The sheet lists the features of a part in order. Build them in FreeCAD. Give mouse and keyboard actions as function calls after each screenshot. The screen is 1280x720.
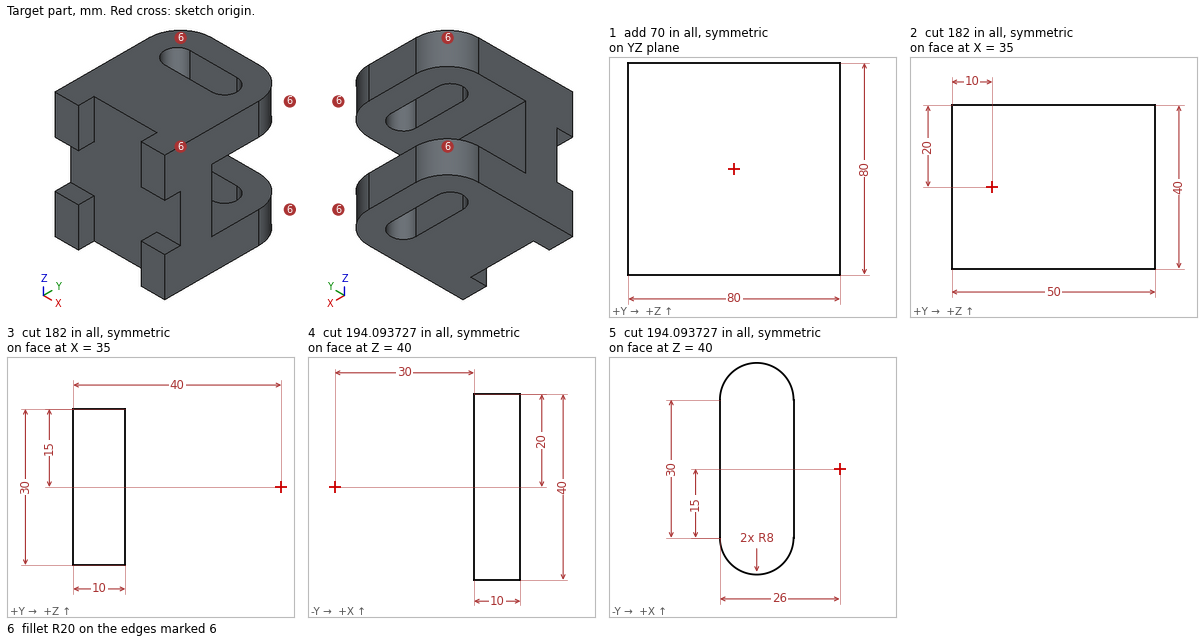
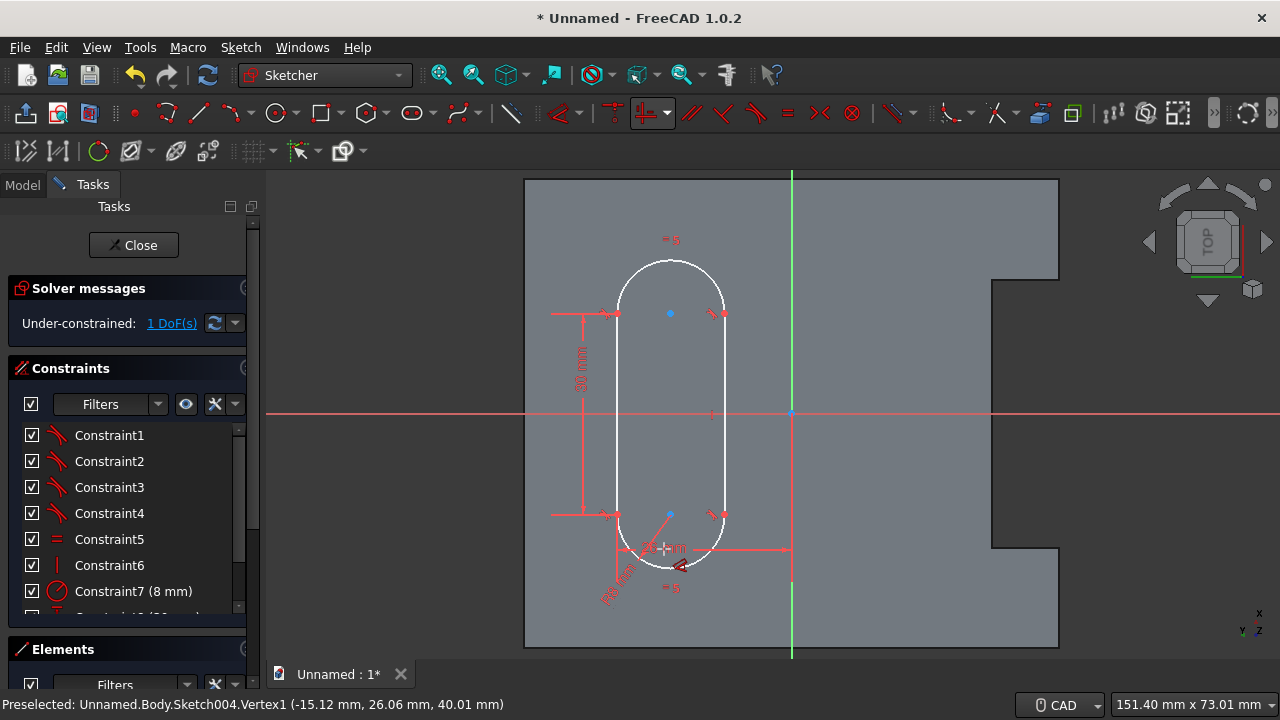
click(617, 515)
click(826, 464)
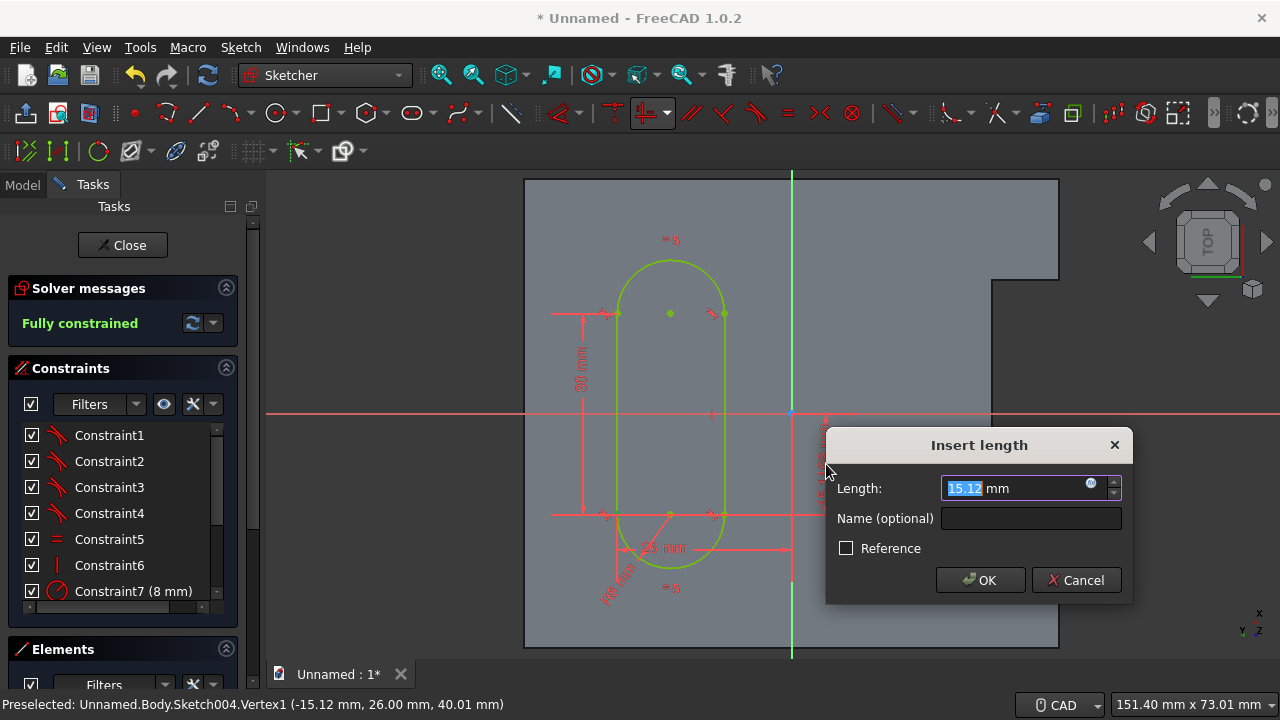
text(15)
key(Return)
key(Escape)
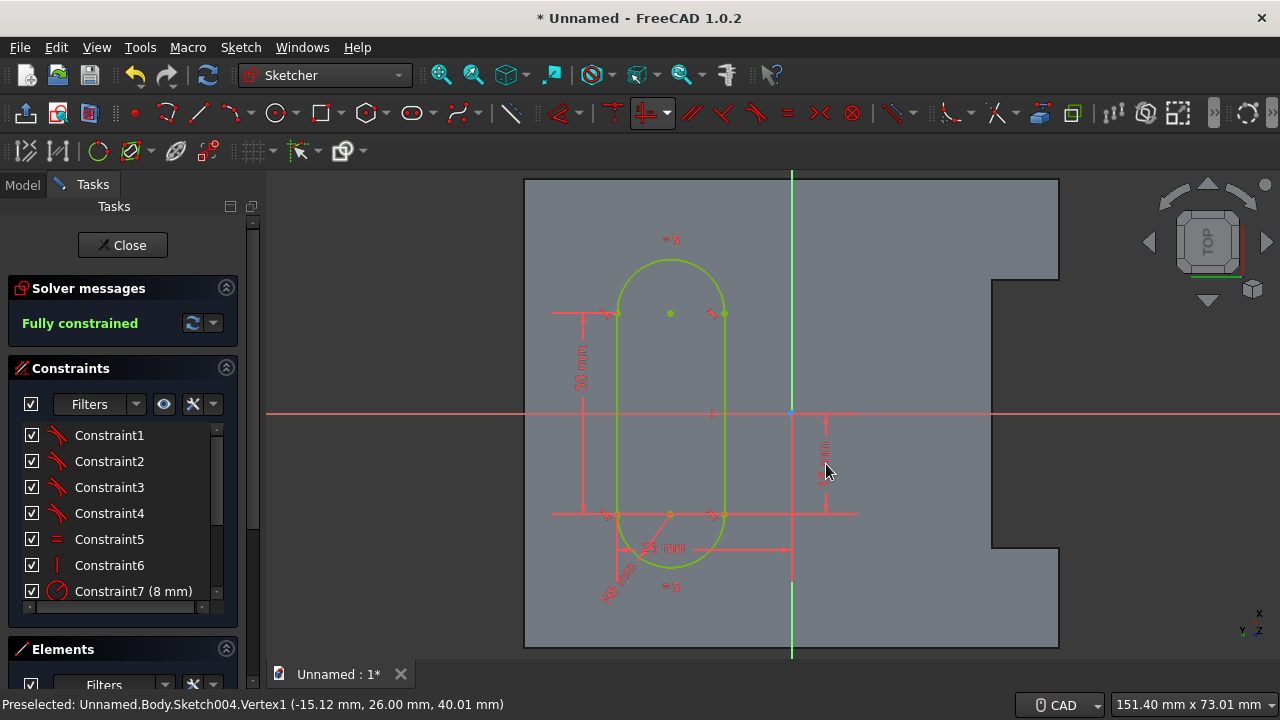
click(123, 245)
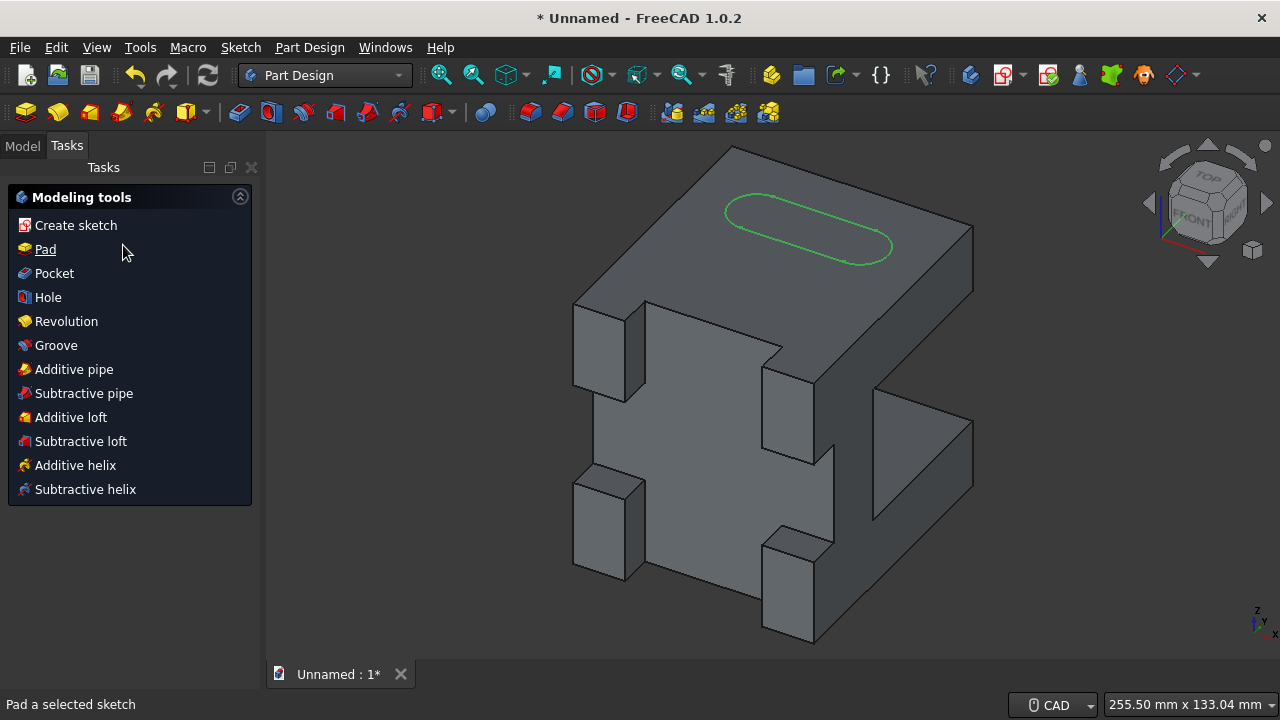
click(240, 112)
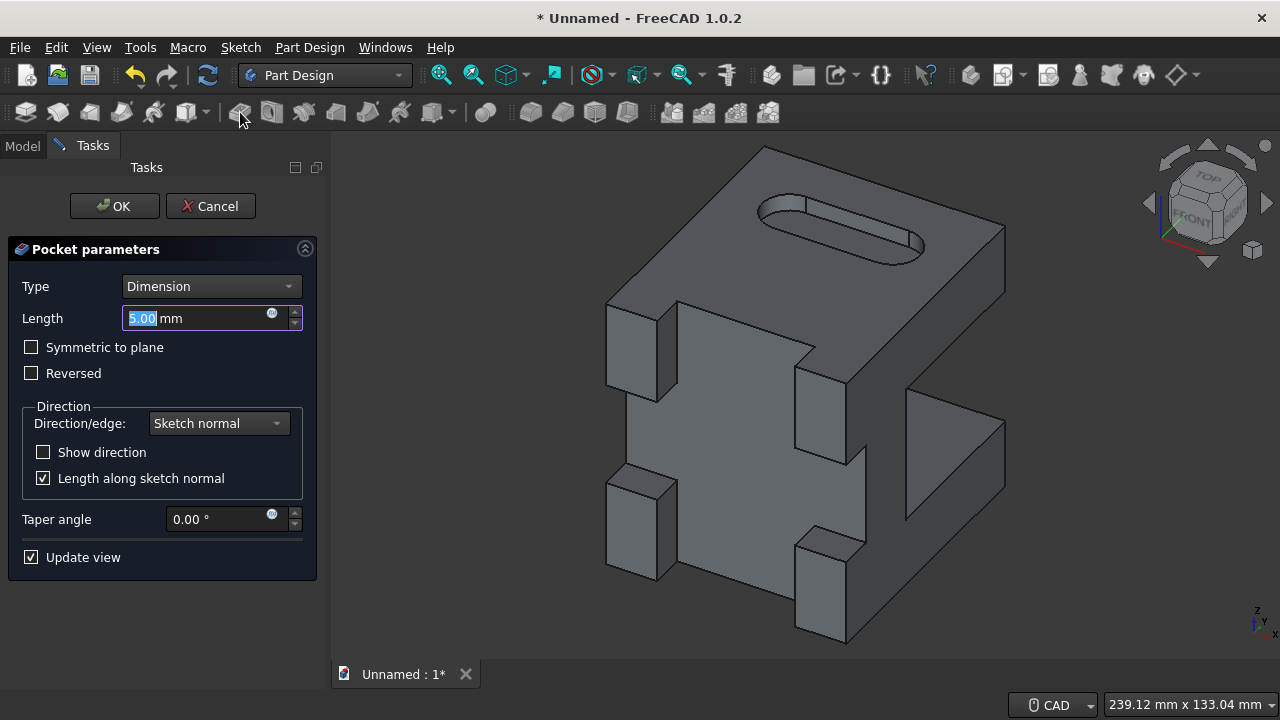
text(194.093727)
key(Tab)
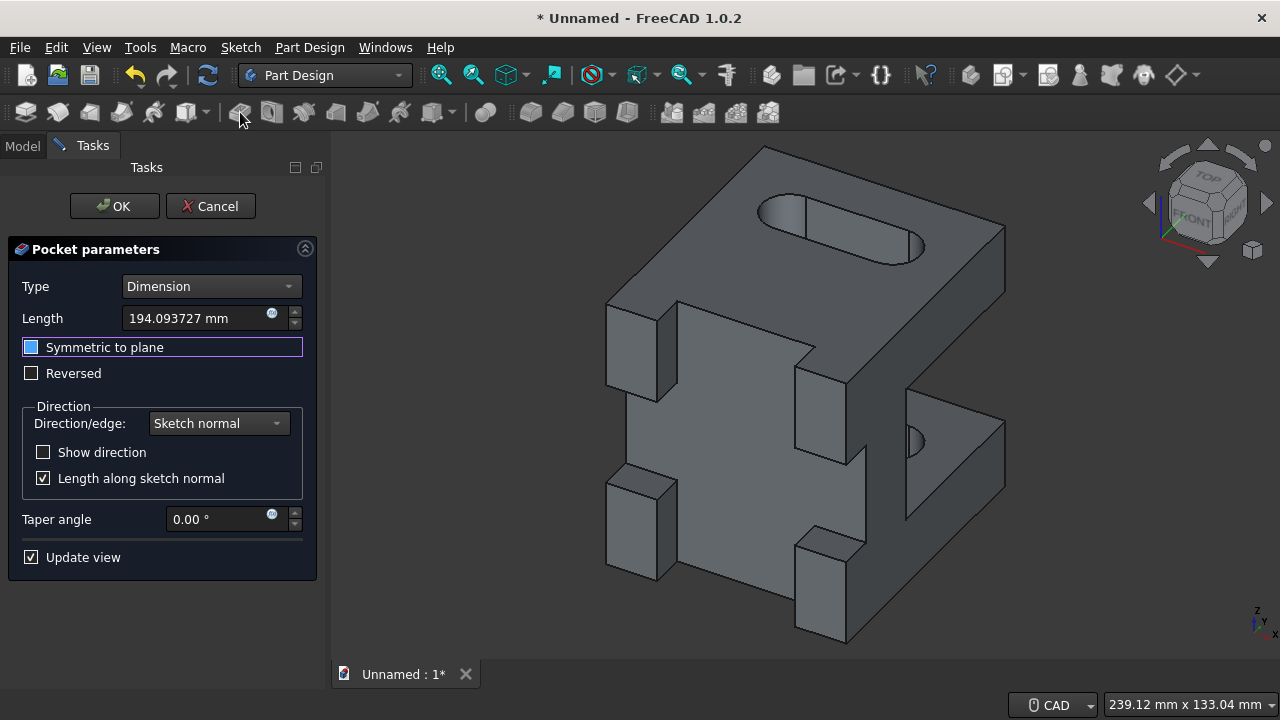
click(30, 347)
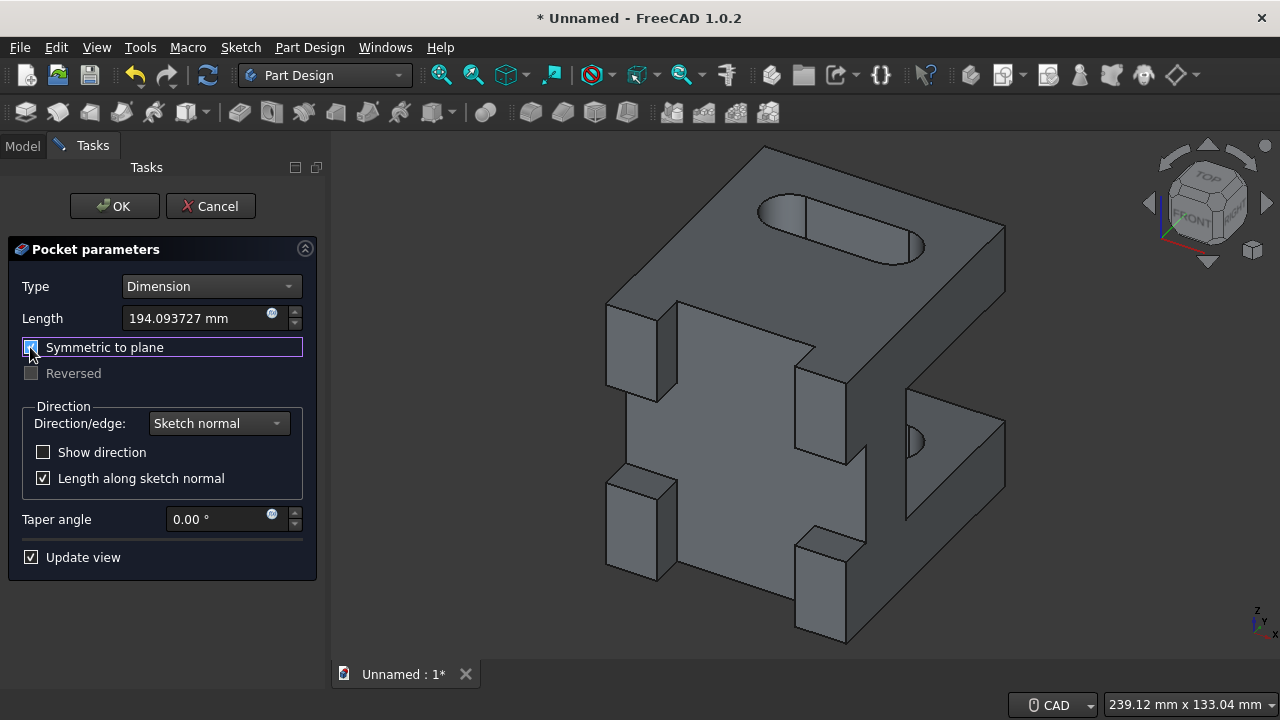
click(115, 206)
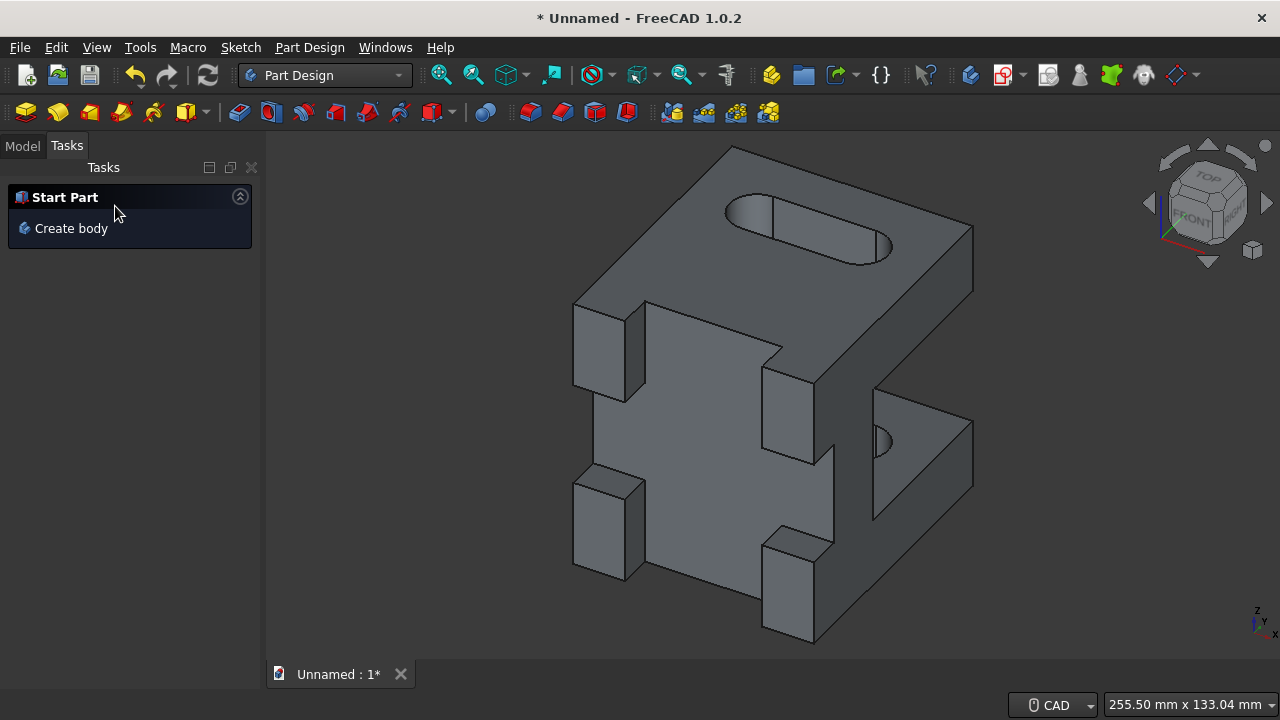
key(0)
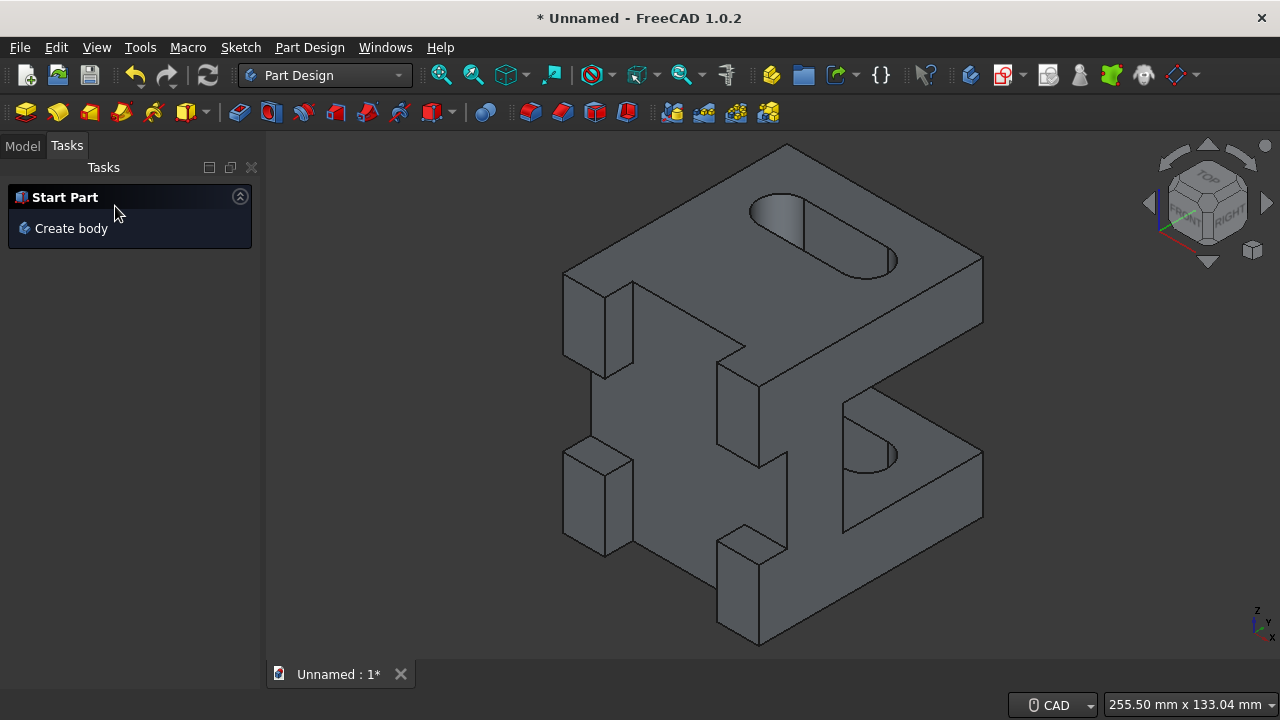
key(2)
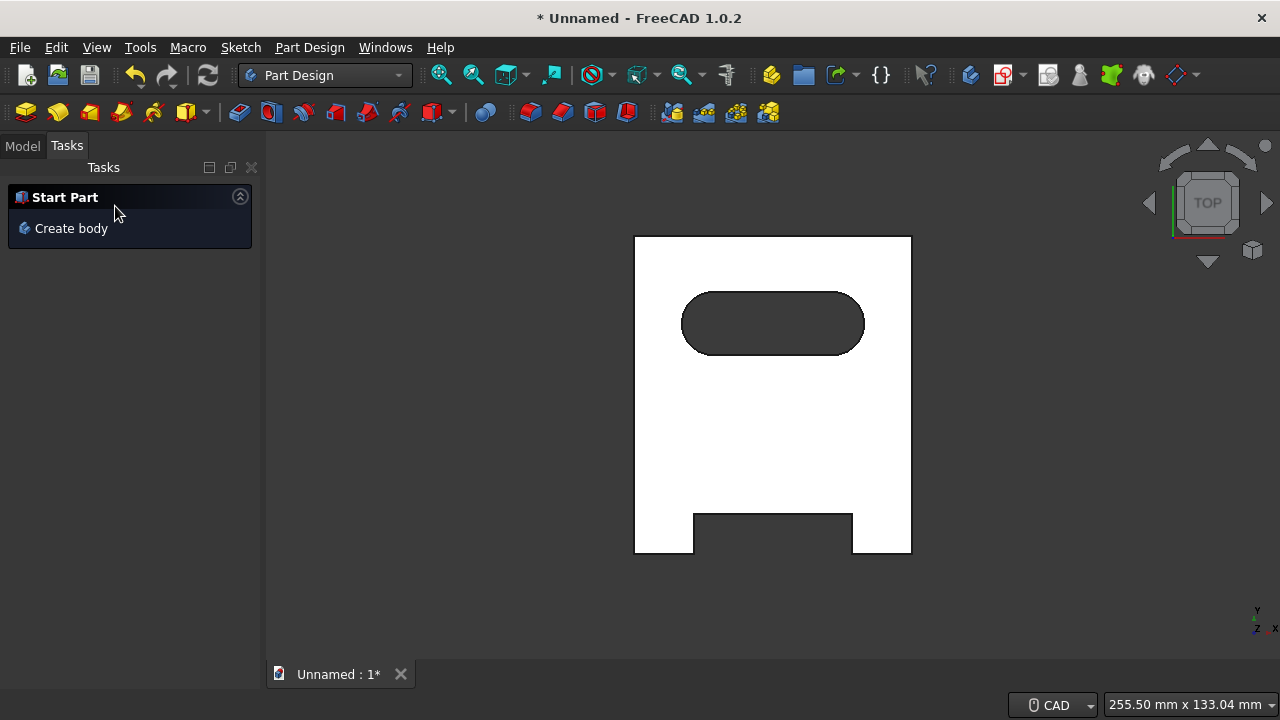
key(1)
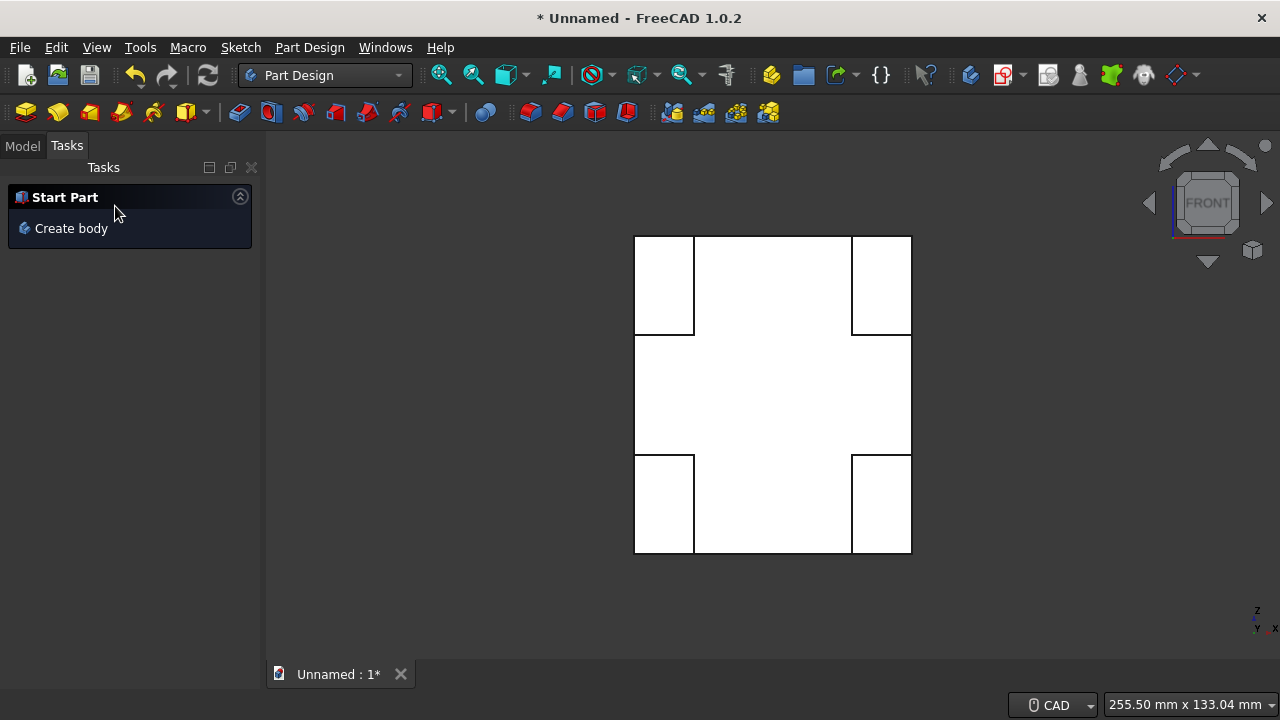
key(3)